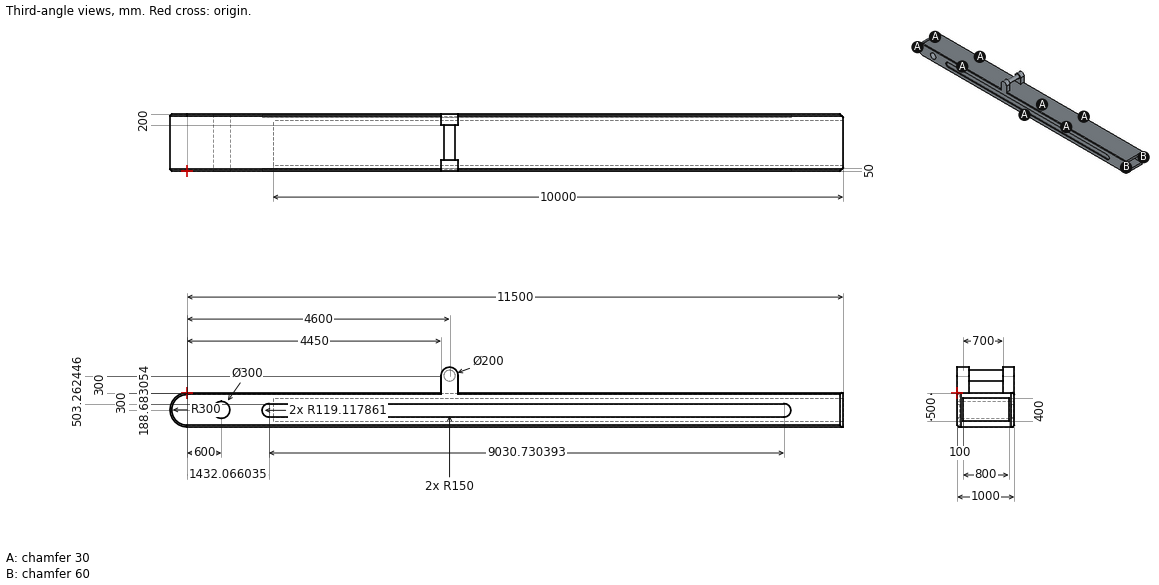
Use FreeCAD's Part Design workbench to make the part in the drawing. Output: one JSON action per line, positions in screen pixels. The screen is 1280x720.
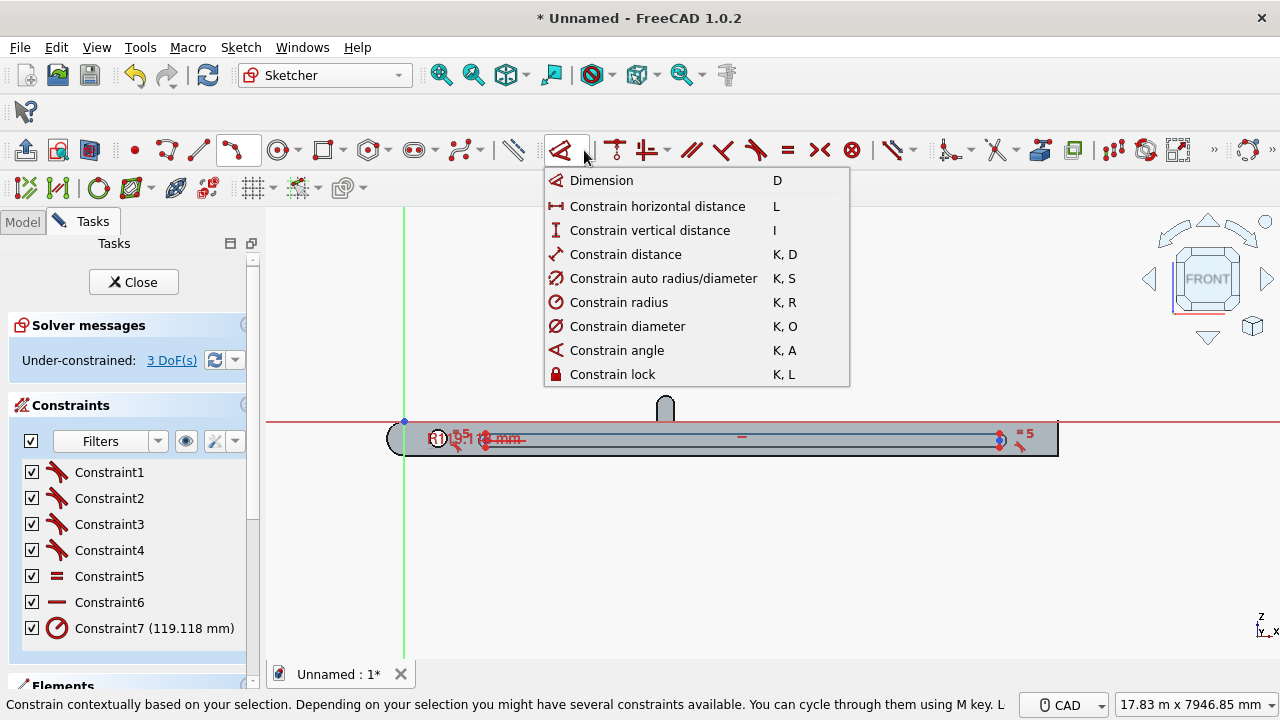
{"action": "left_click", "coordinate": [697, 206]}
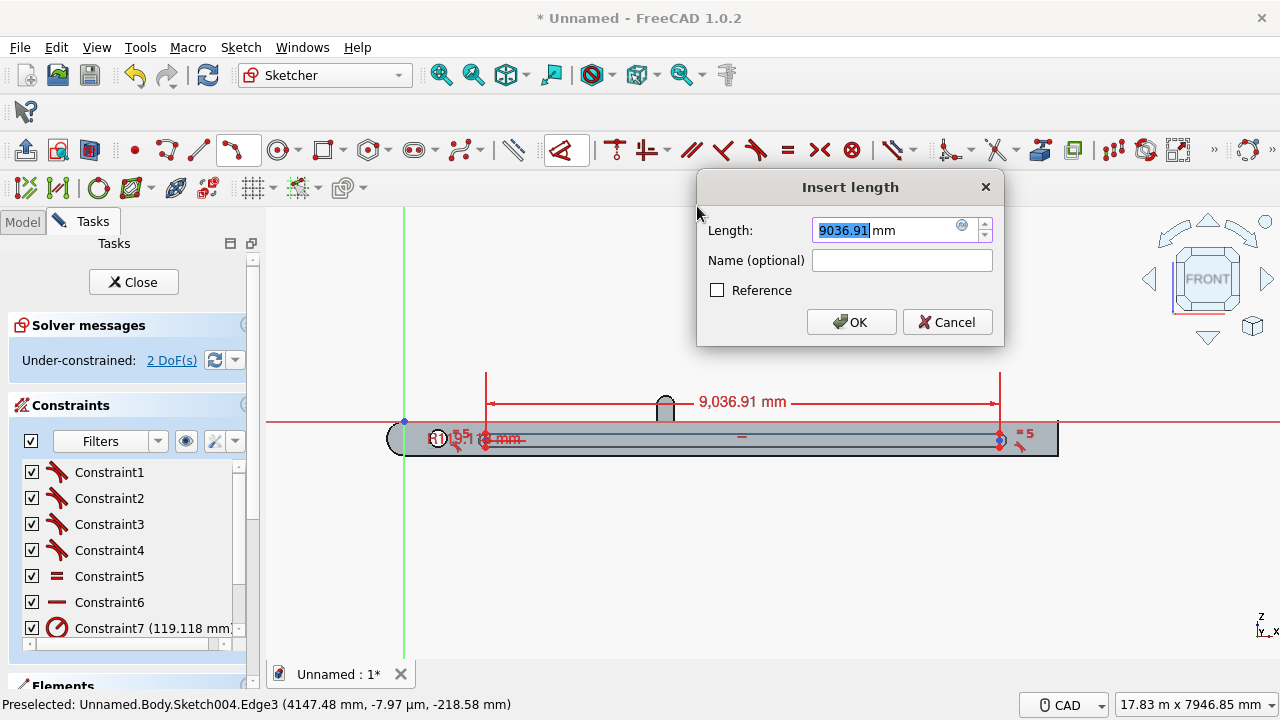
{"action": "type", "text": "9030.730393"}
{"action": "key", "text": "Return"}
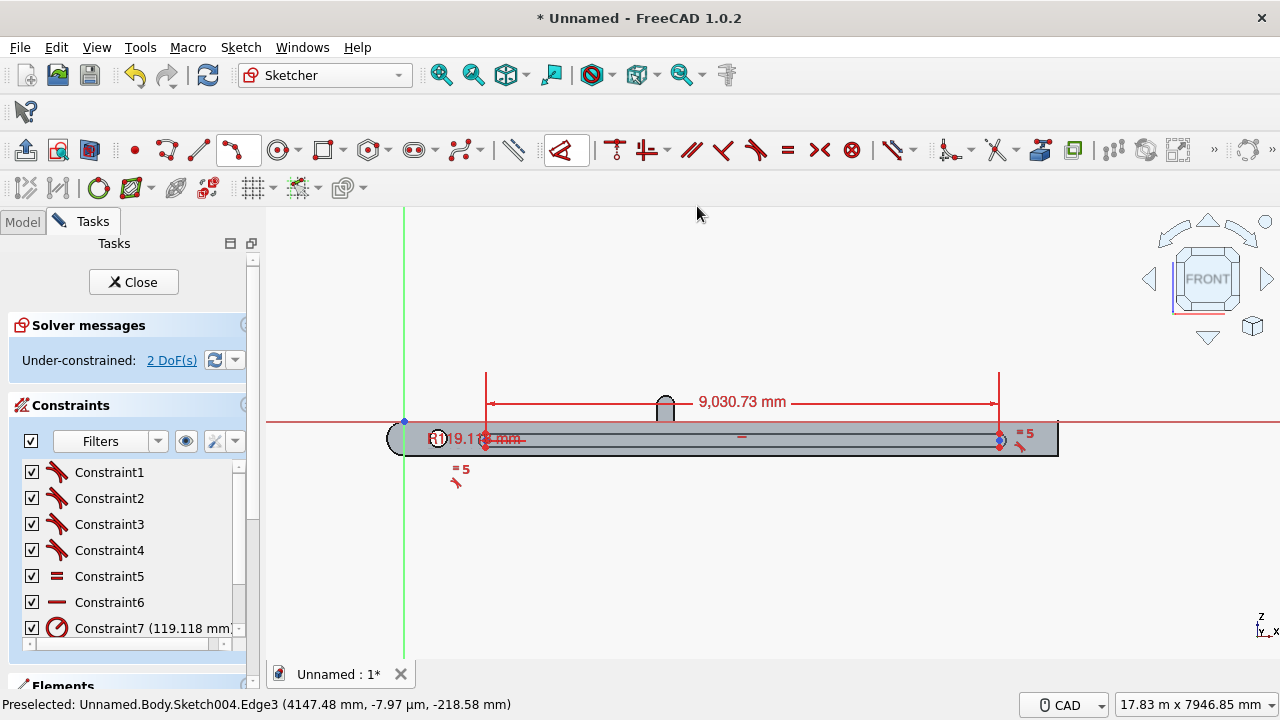
{"action": "scroll", "coordinate": [486, 434], "scroll_direction": "up", "scroll_amount": 7}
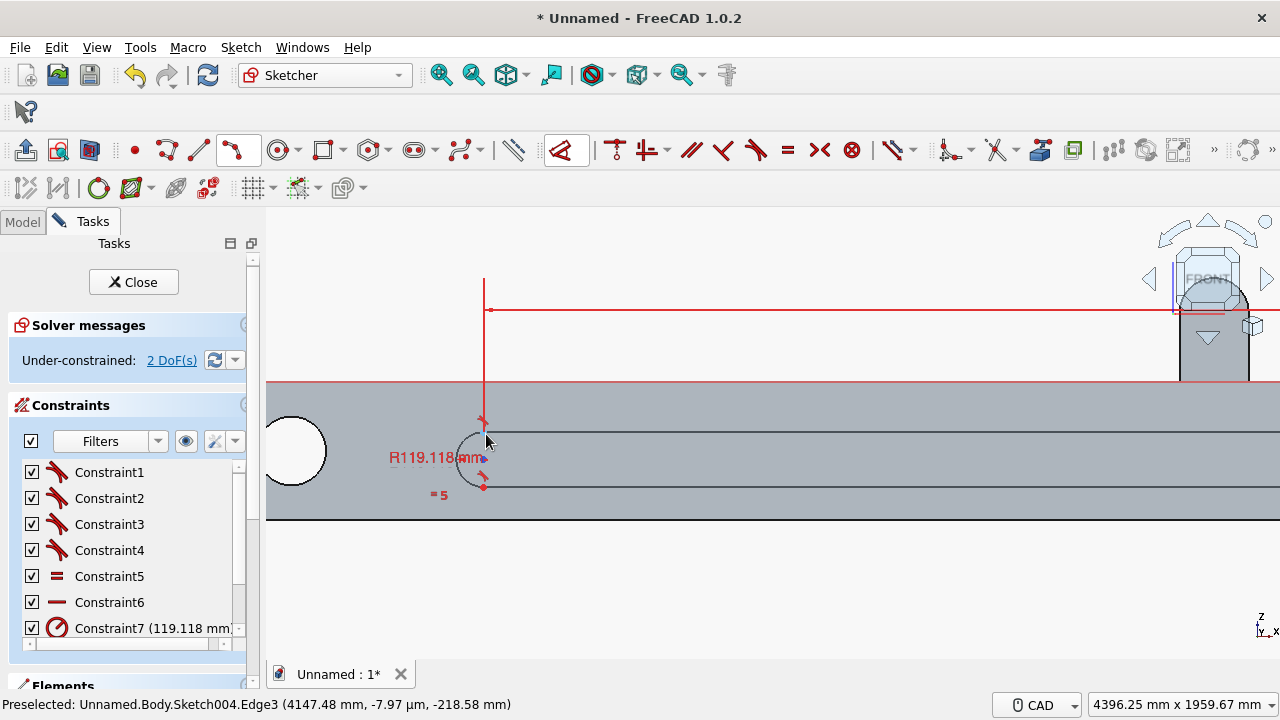
{"action": "left_click", "coordinate": [484, 432]}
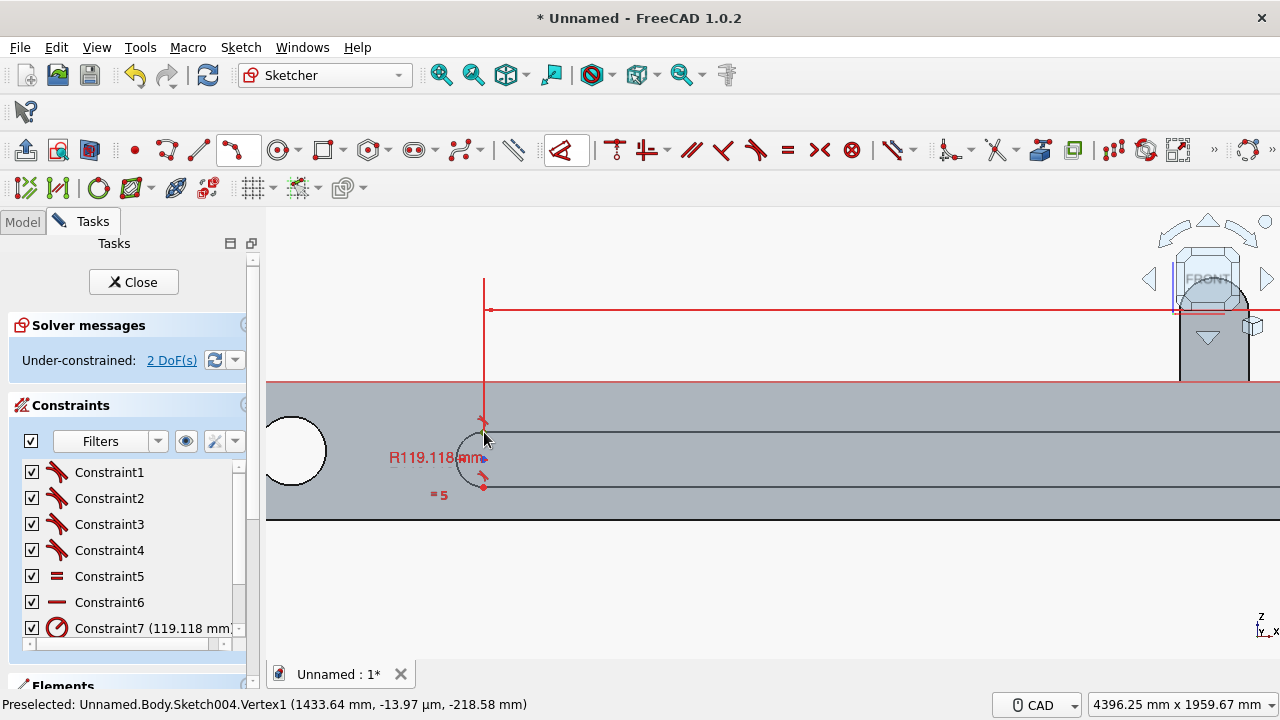
{"action": "key", "text": "i"}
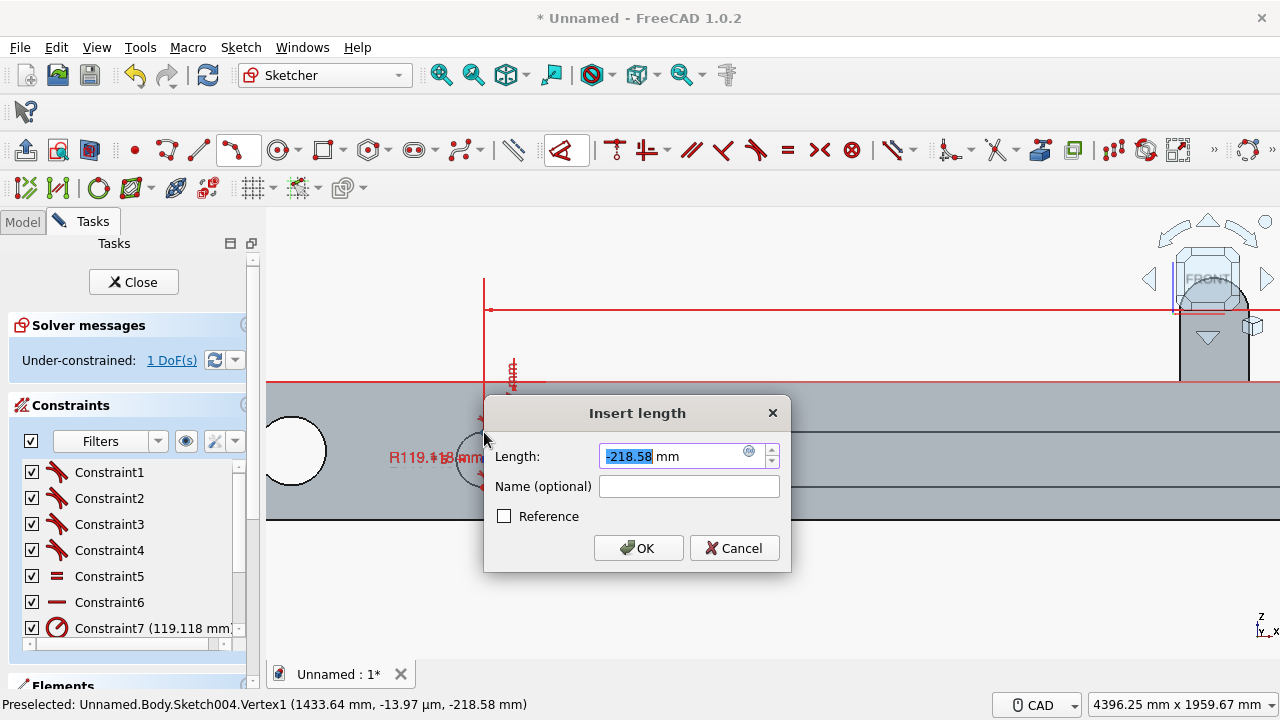
{"action": "type", "text": "-188.683054"}
{"action": "key", "text": "Return"}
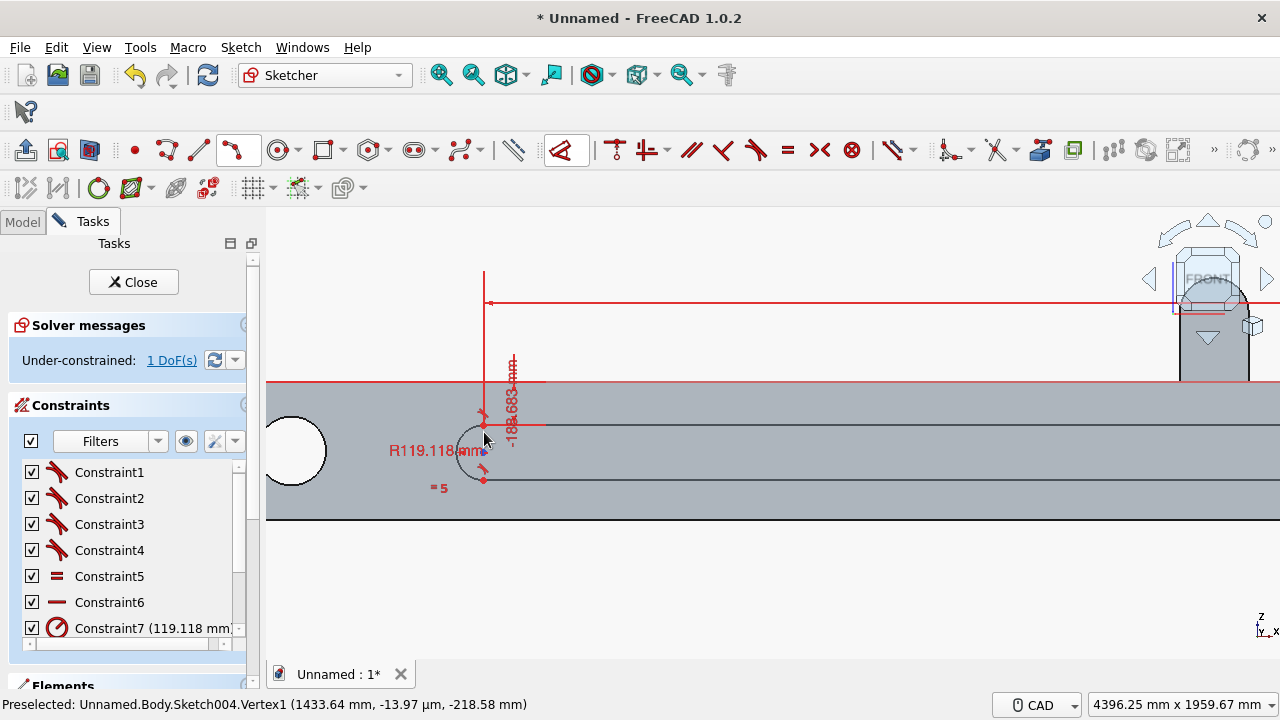
{"action": "left_click", "coordinate": [484, 425]}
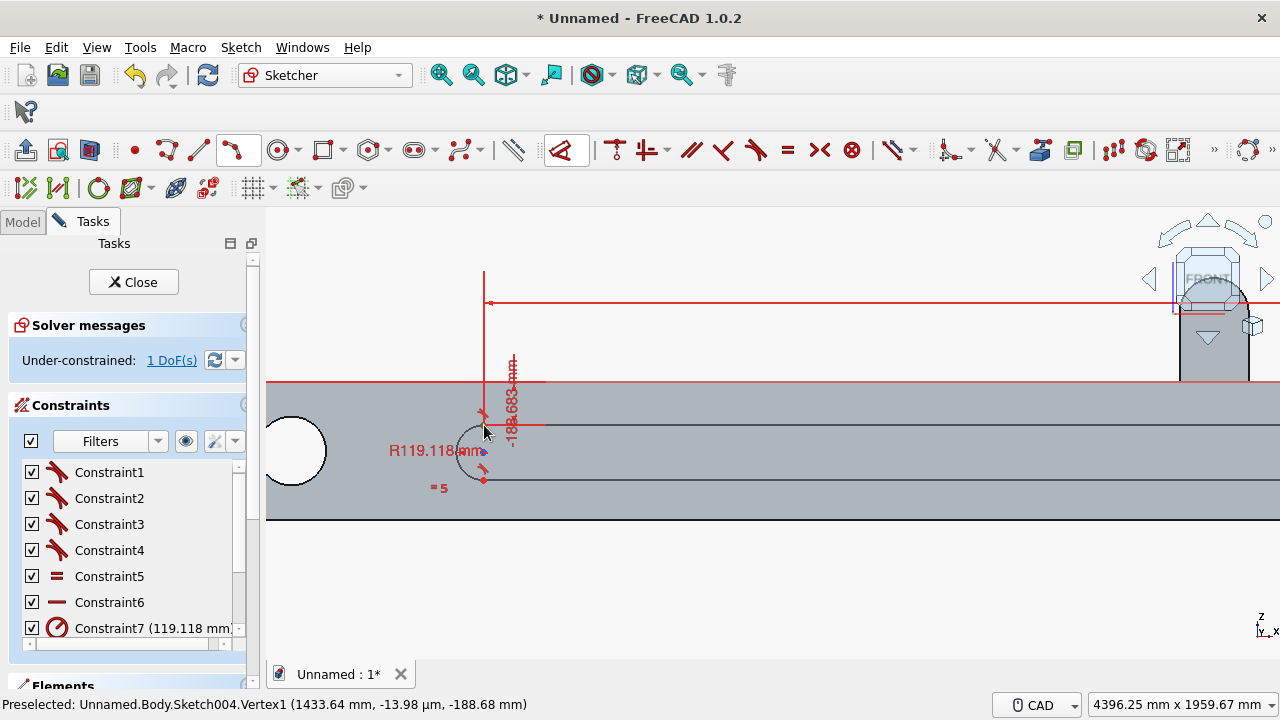
{"action": "left_click", "coordinate": [584, 150]}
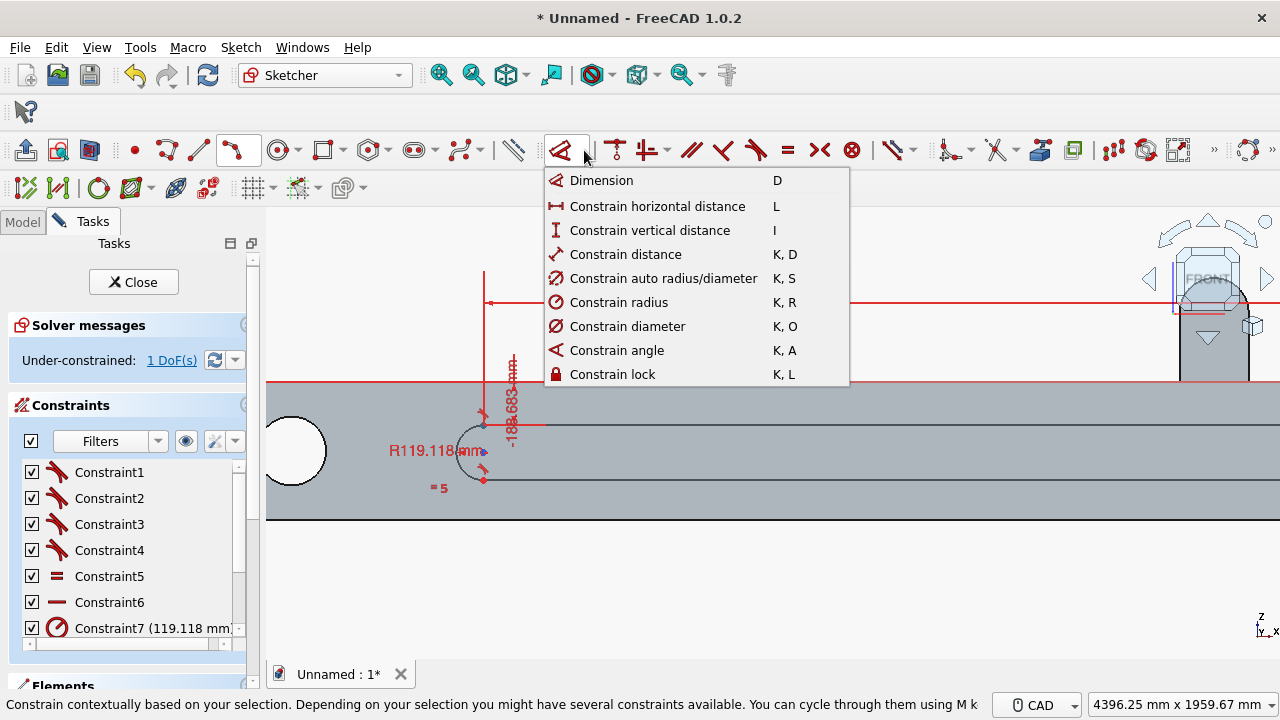
{"action": "left_click", "coordinate": [697, 206]}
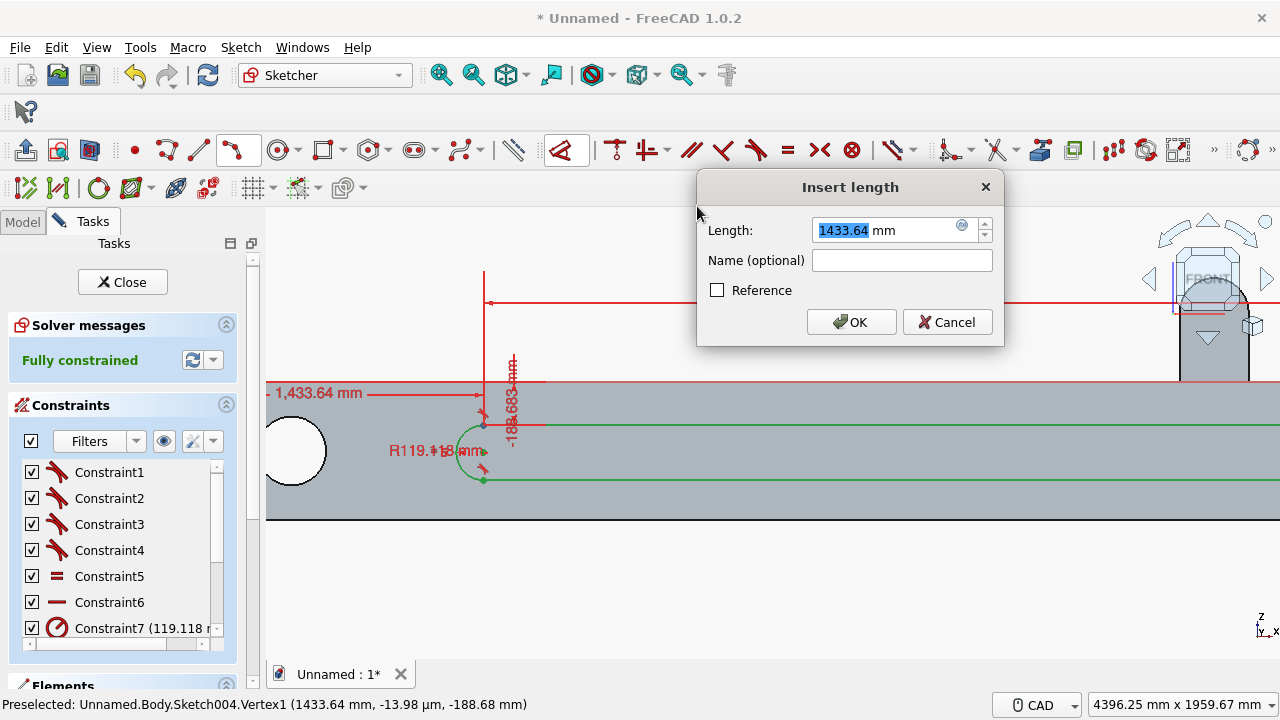
{"action": "type", "text": "1432.066035"}
{"action": "key", "text": "Return"}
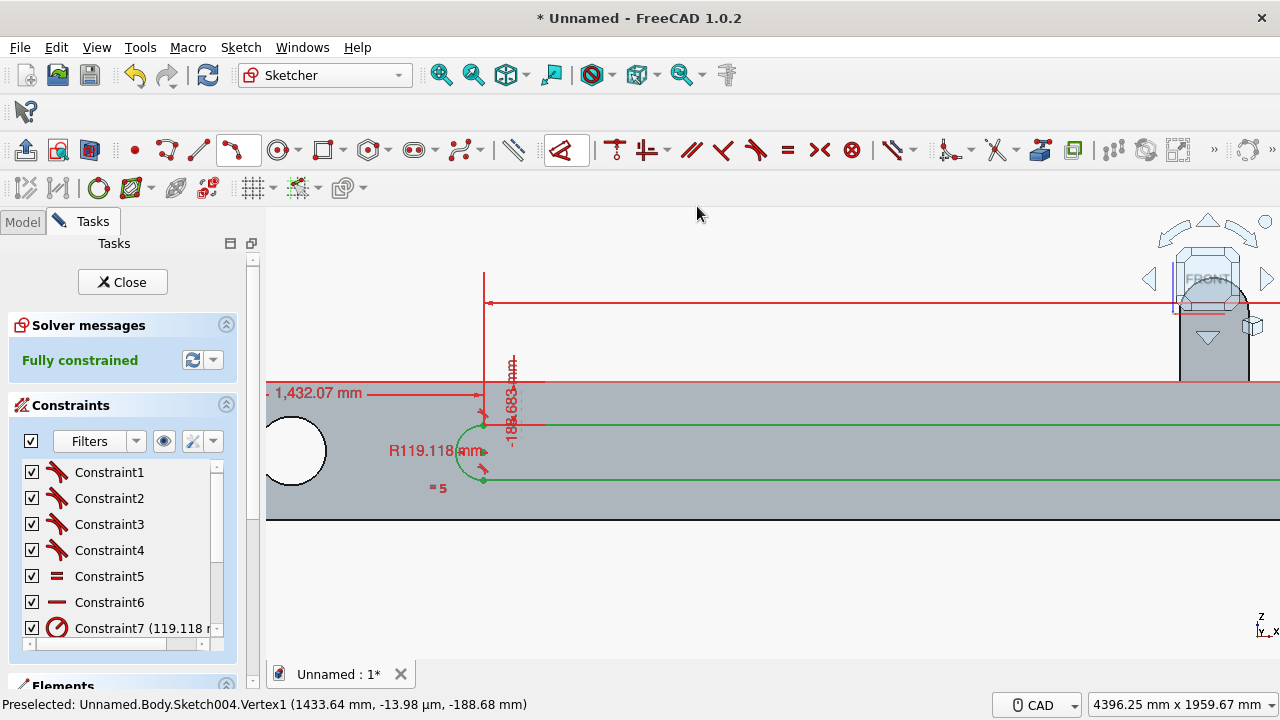
{"action": "left_click", "coordinate": [123, 282]}